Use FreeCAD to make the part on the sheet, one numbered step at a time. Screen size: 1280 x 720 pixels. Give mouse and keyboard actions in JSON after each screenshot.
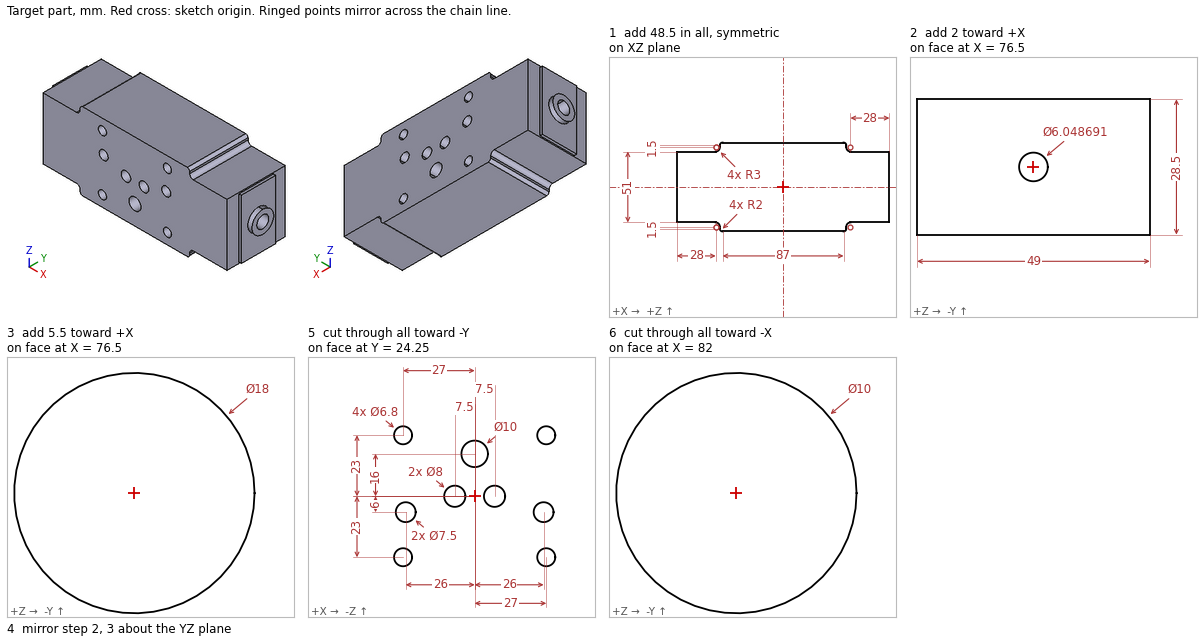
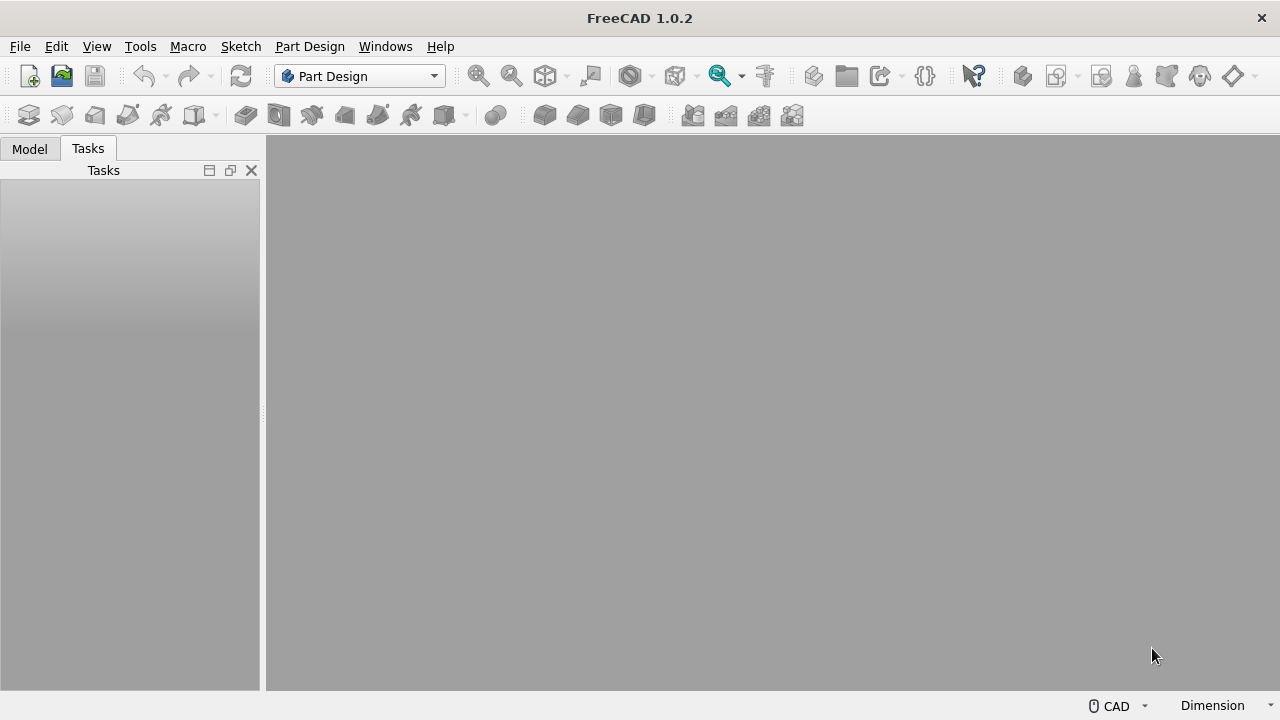
{"action": "left_click", "coordinate": [29, 76]}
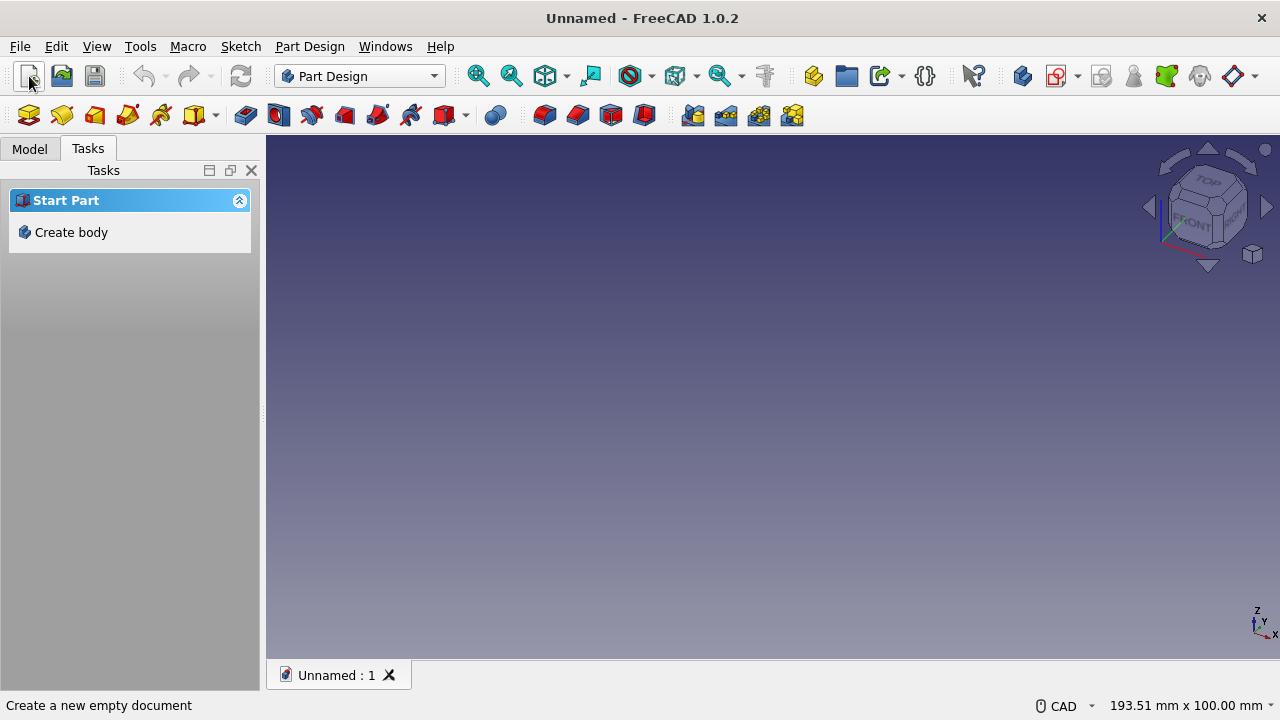
{"action": "left_click", "coordinate": [1056, 76]}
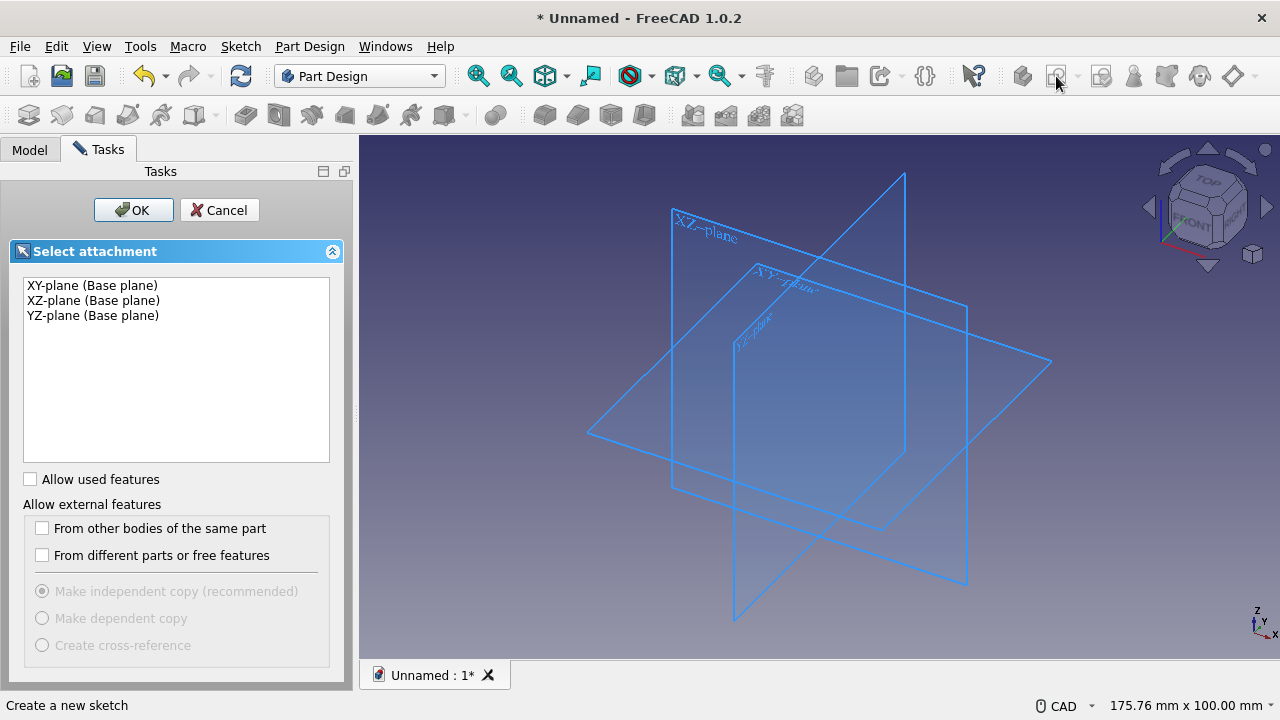
{"action": "left_click", "coordinate": [84, 300]}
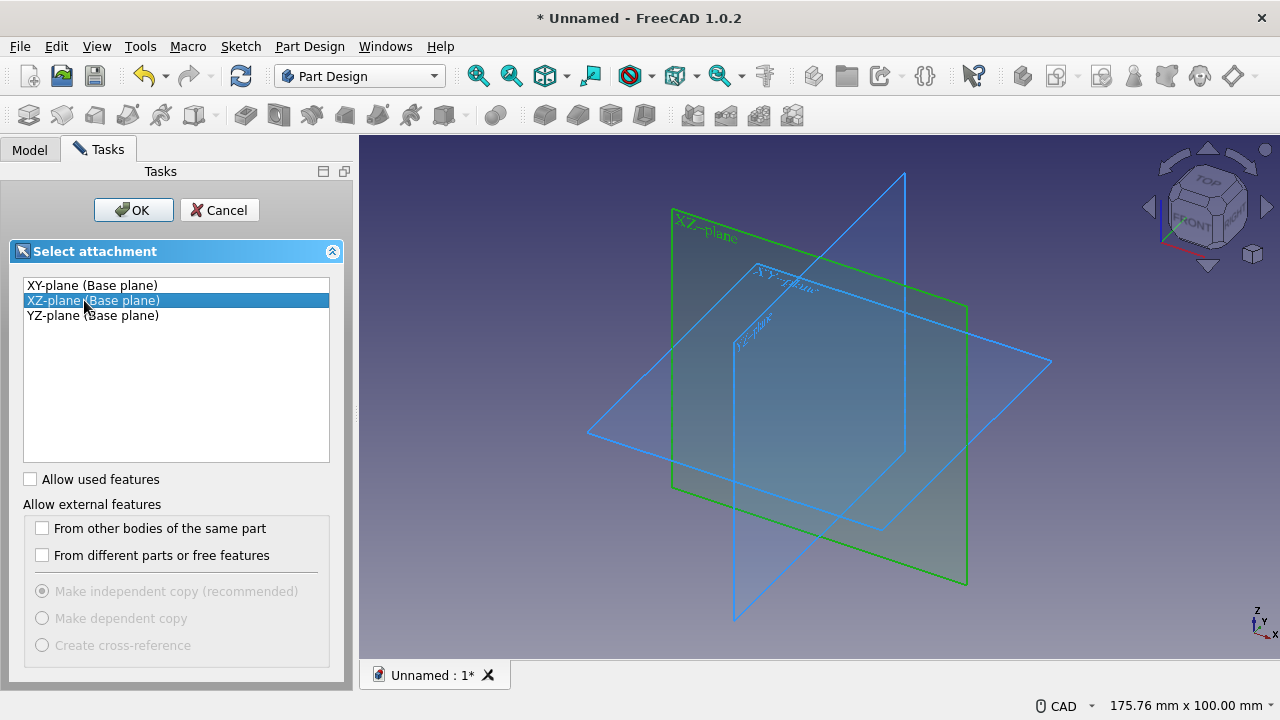
{"action": "left_click", "coordinate": [134, 210]}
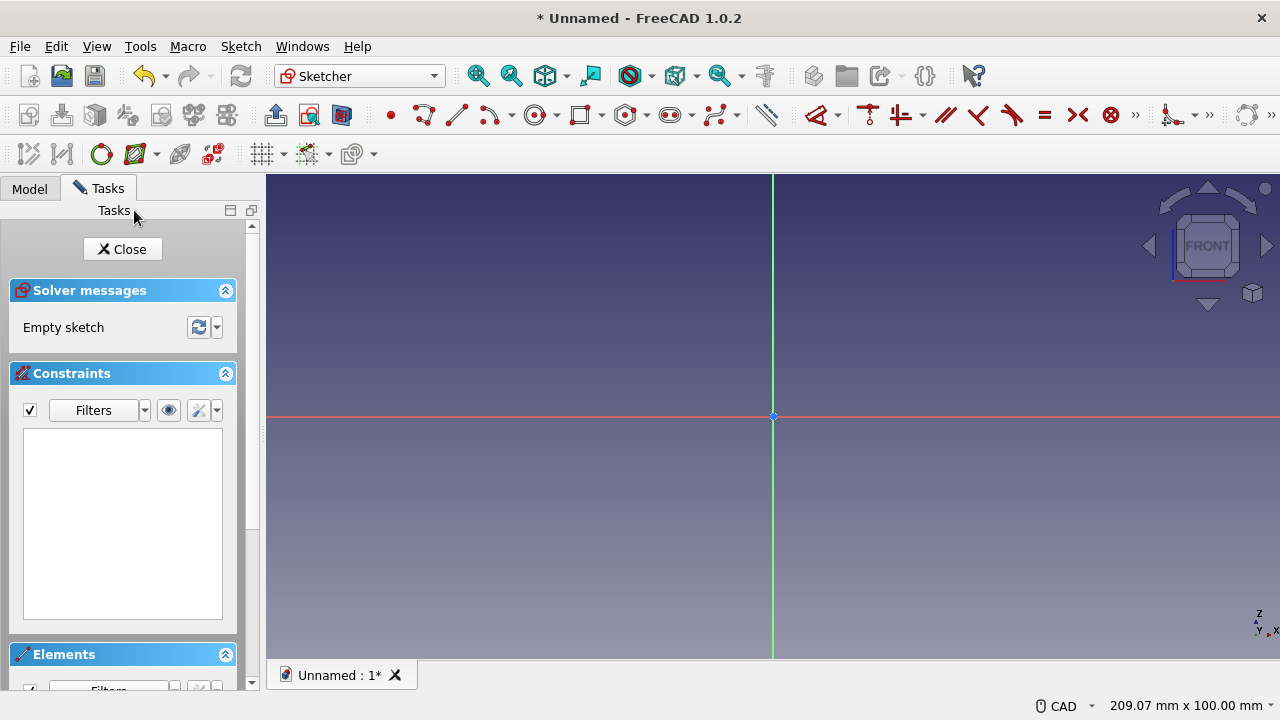
{"action": "scroll", "coordinate": [395, 416], "scroll_direction": "down", "scroll_amount": 1}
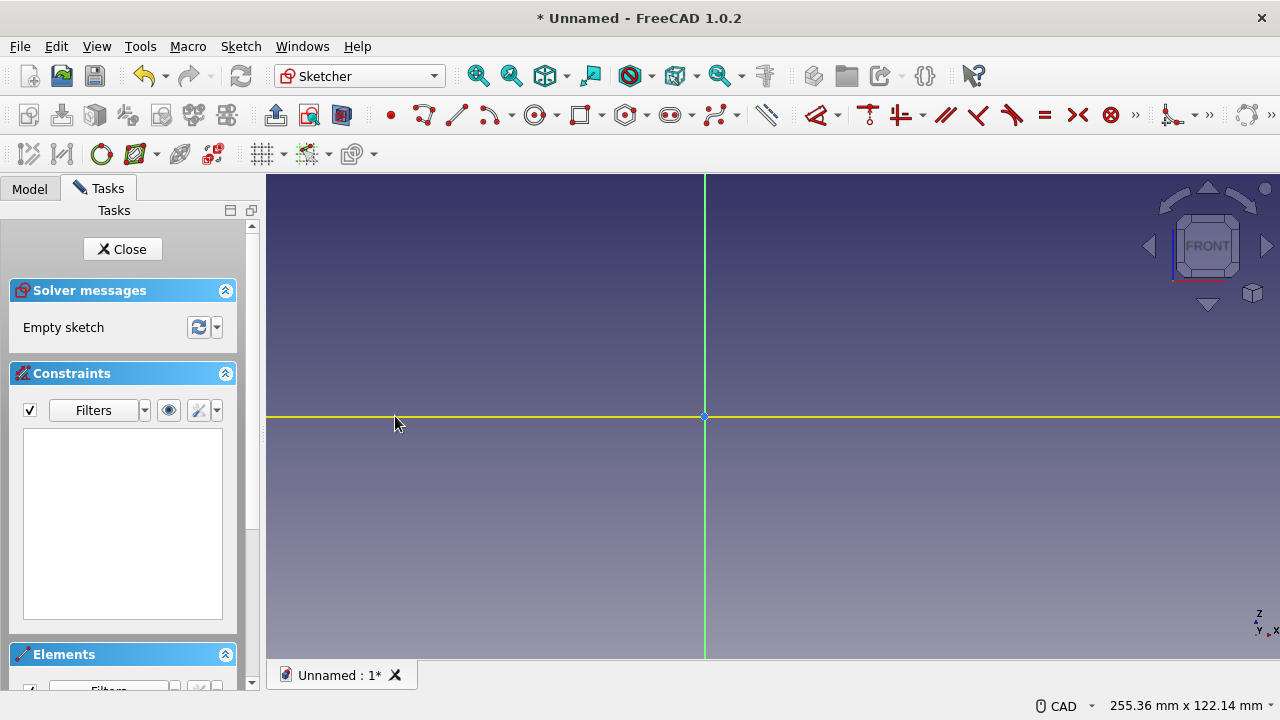
{"action": "left_click", "coordinate": [457, 116]}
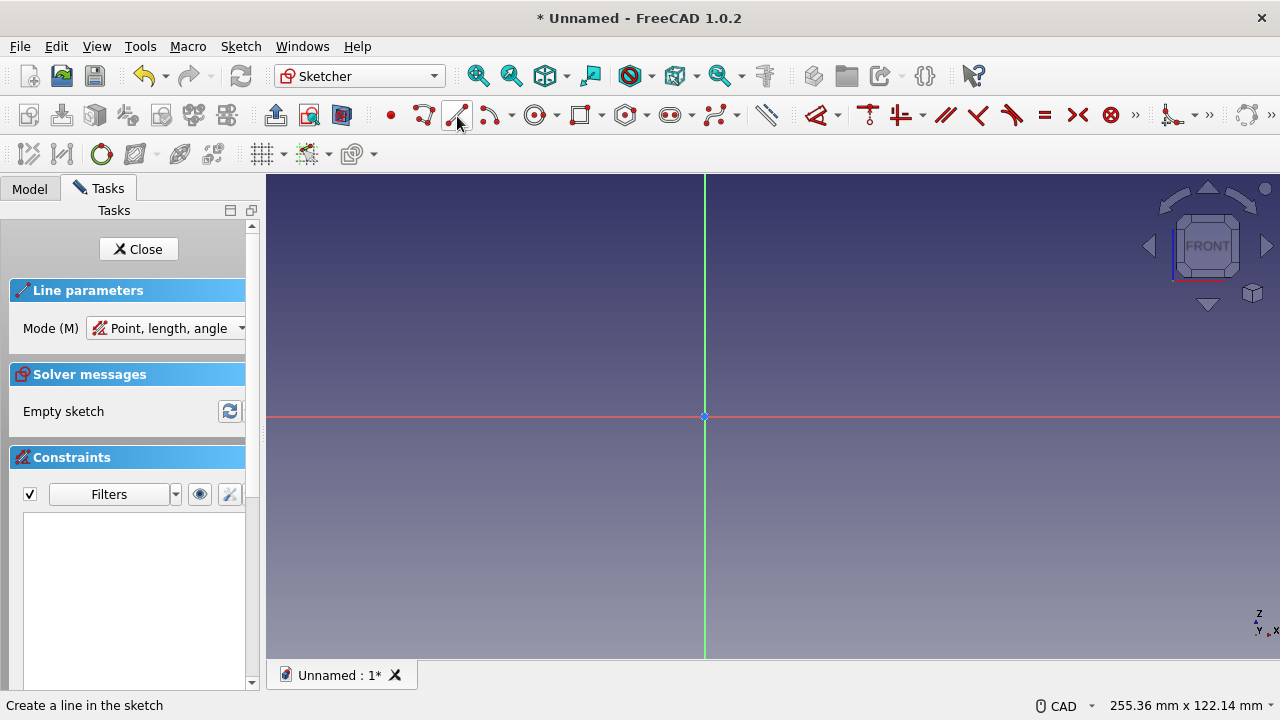
{"action": "left_click", "coordinate": [877, 544]}
{"action": "left_click", "coordinate": [532, 544]}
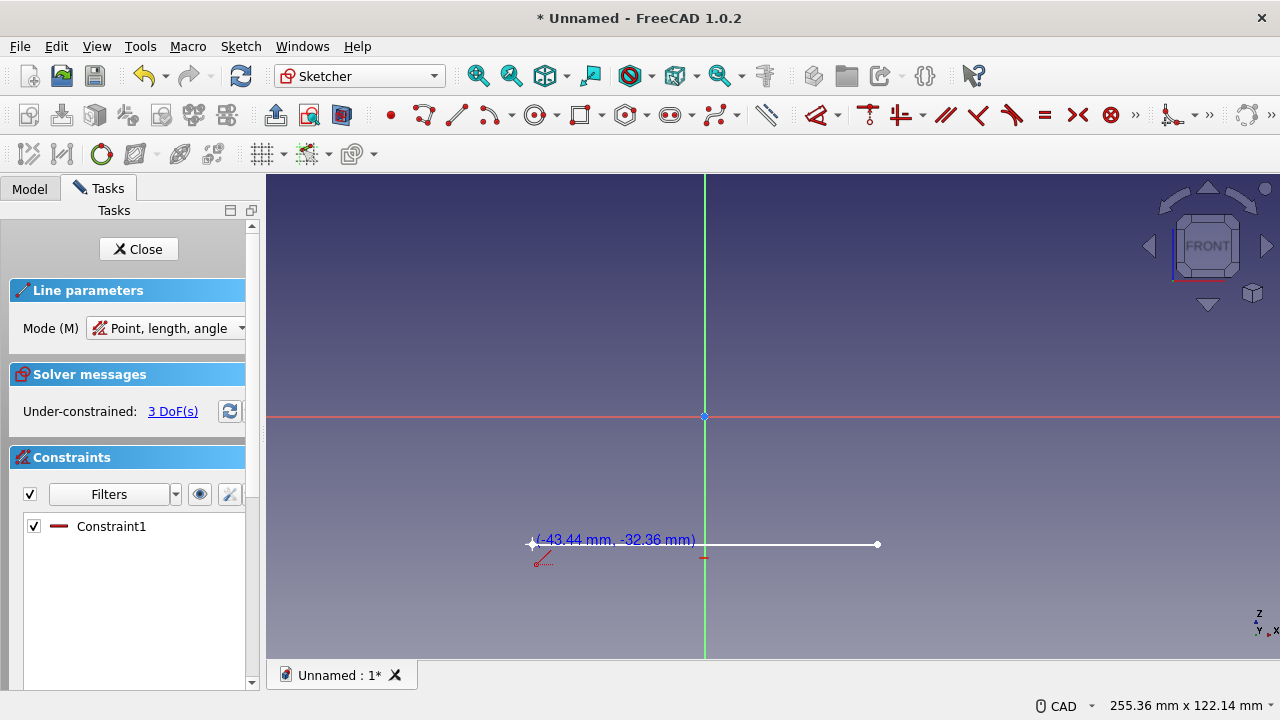
{"action": "scroll", "coordinate": [524, 536], "scroll_direction": "up", "scroll_amount": 2}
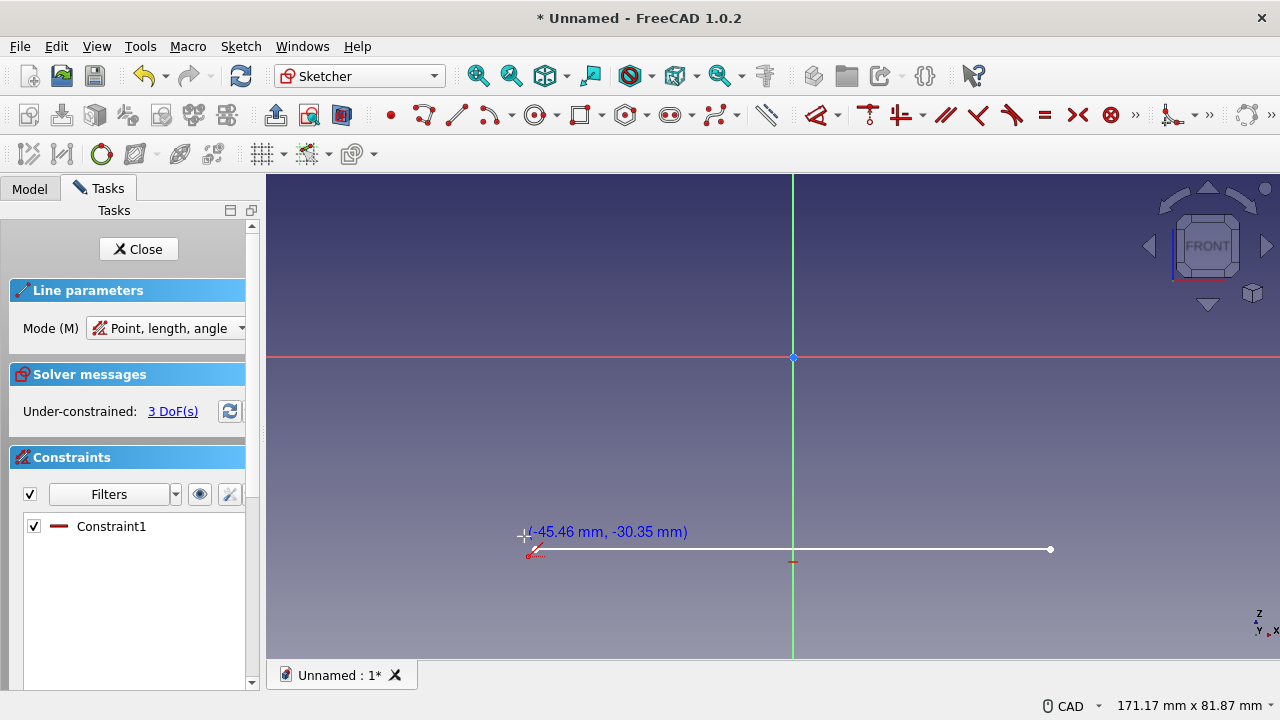
{"action": "left_click", "coordinate": [524, 535]}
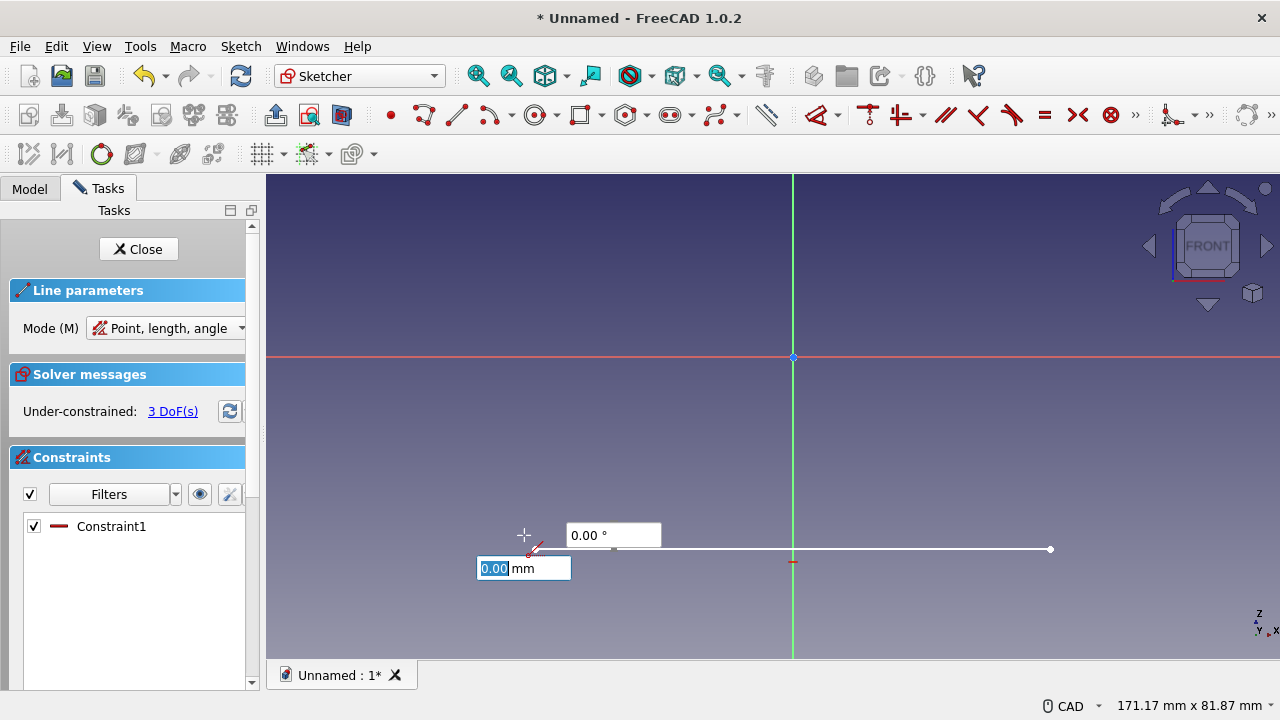
{"action": "scroll", "coordinate": [524, 526], "scroll_direction": "up", "scroll_amount": 3}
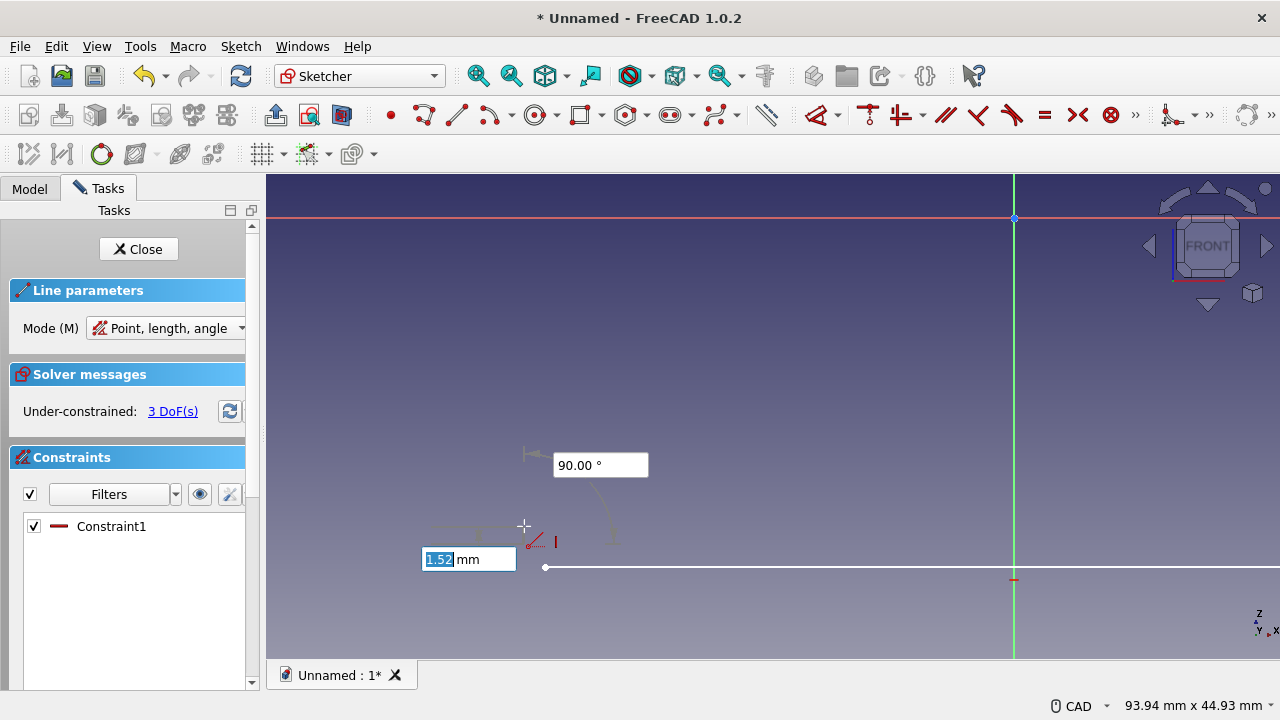
{"action": "left_click", "coordinate": [524, 526]}